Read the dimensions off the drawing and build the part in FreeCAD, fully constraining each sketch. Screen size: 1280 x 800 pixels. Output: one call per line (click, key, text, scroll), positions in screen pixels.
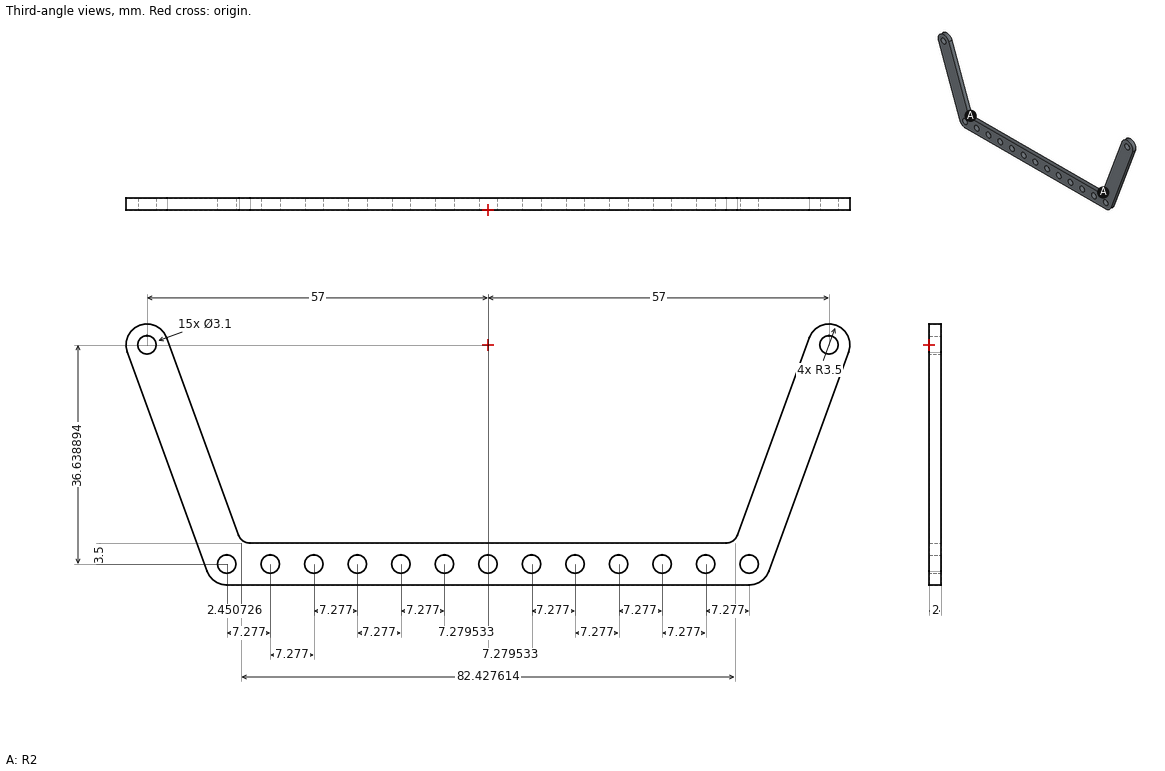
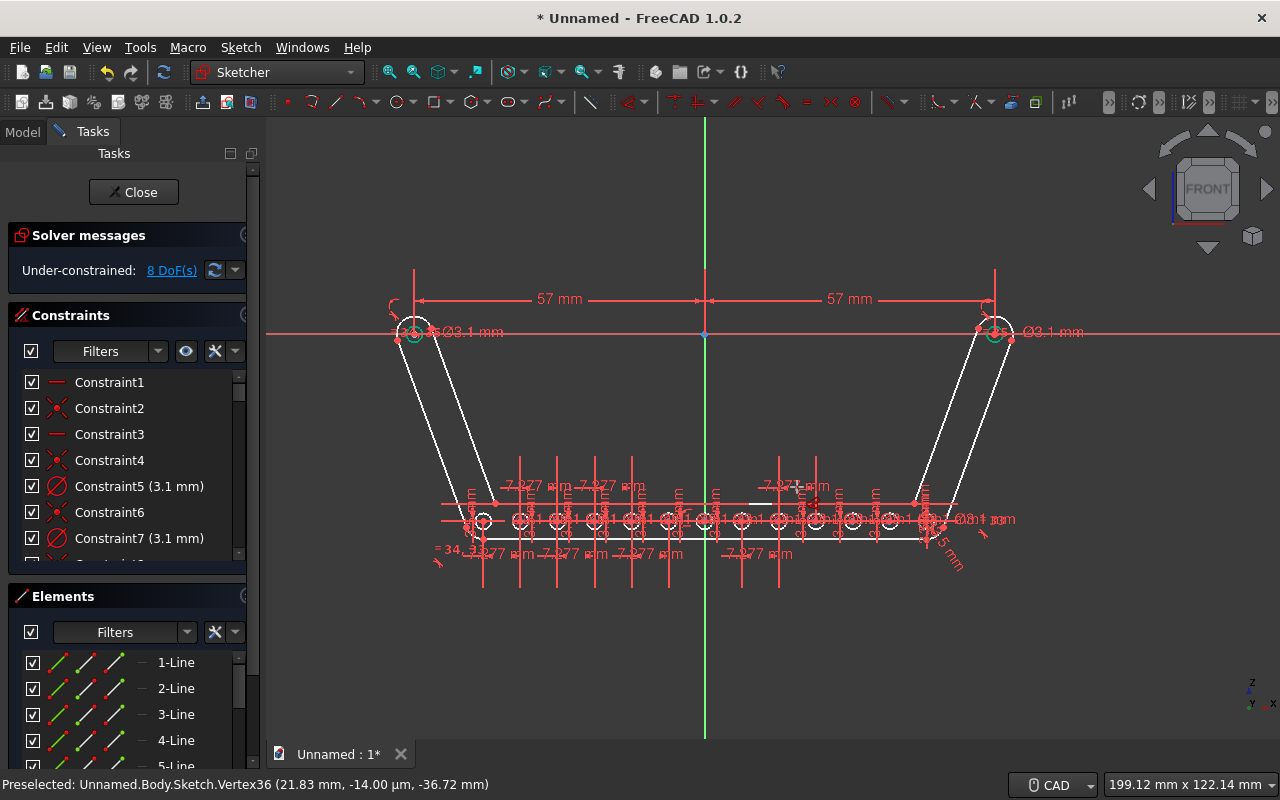
click(816, 521)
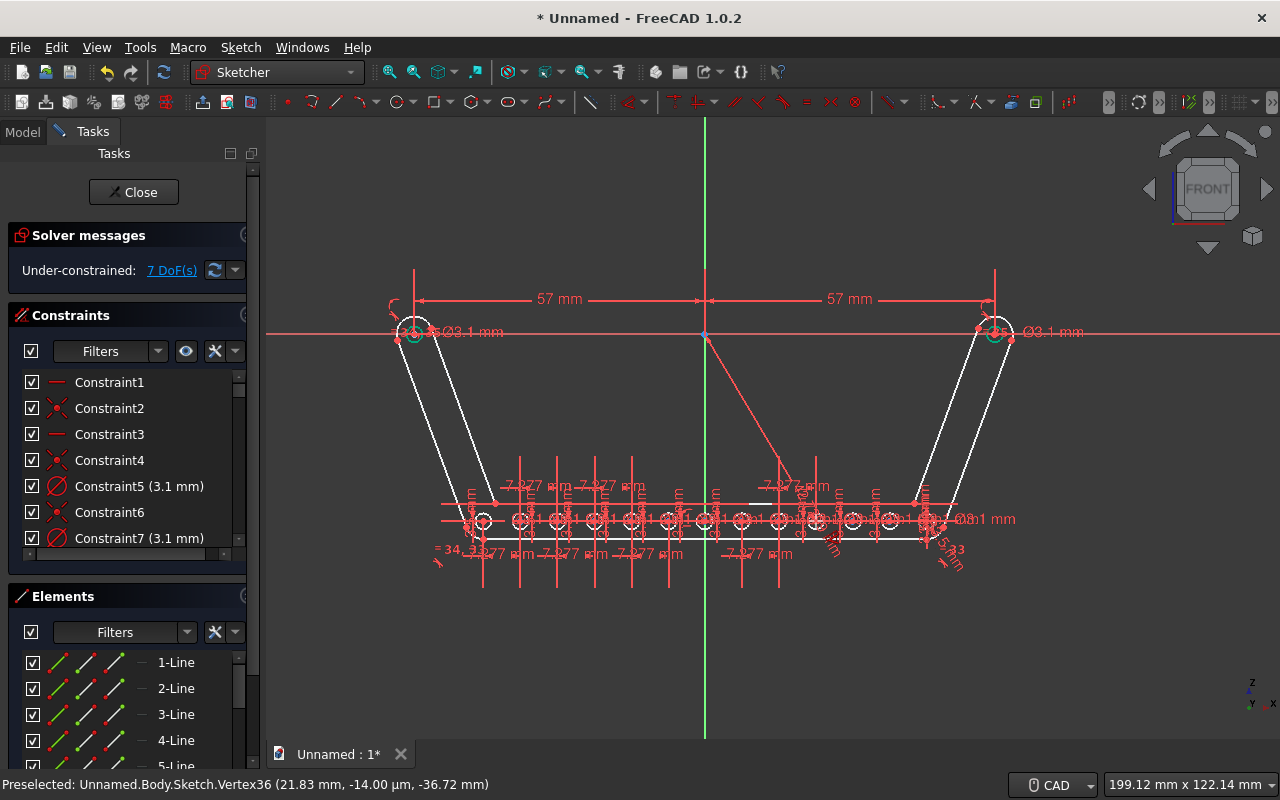
click(853, 521)
click(834, 555)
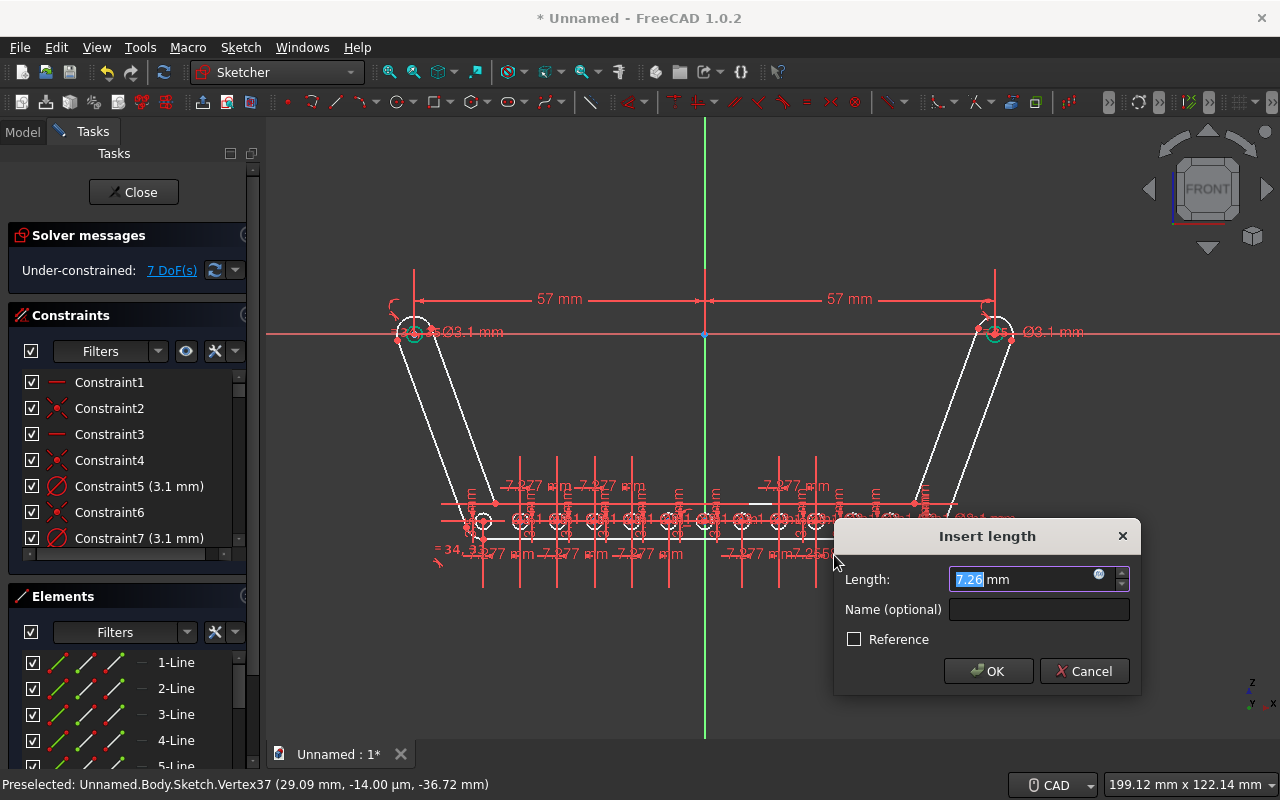
text(7.277)
key(Return)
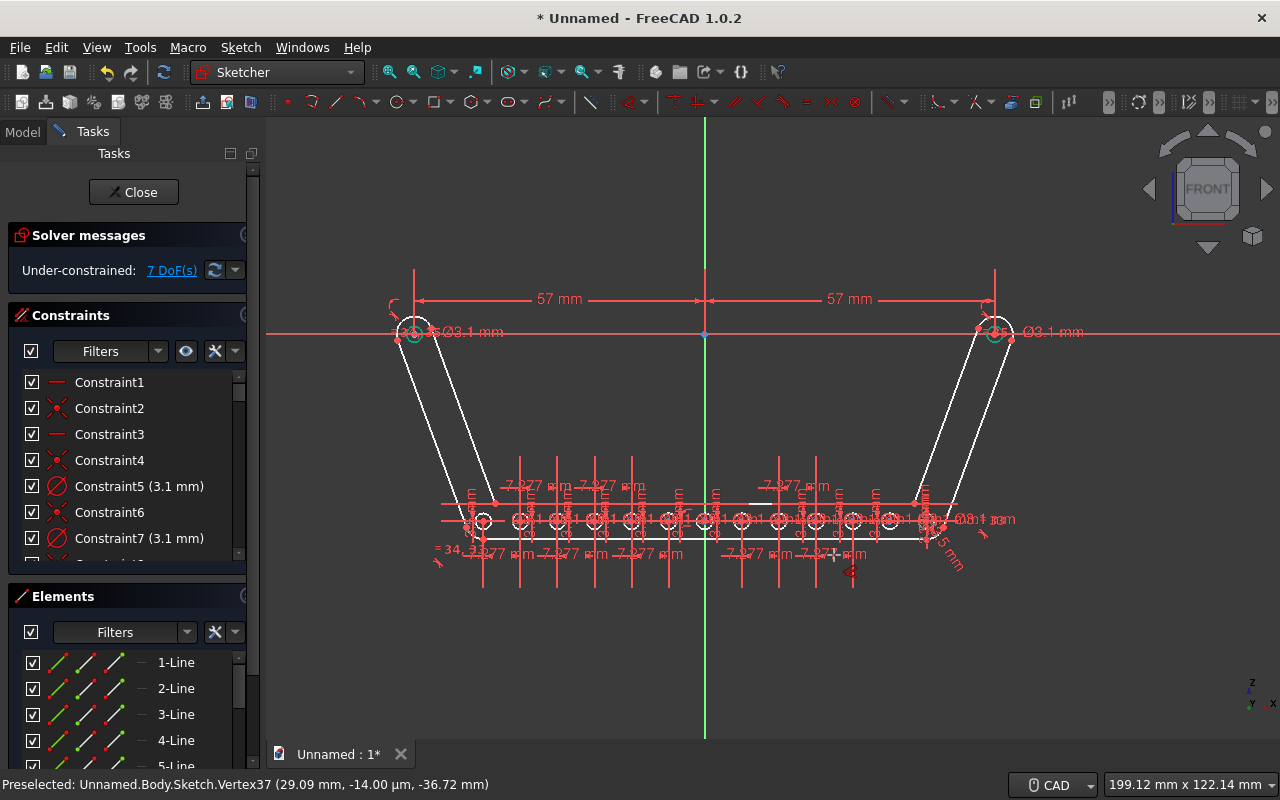
click(853, 521)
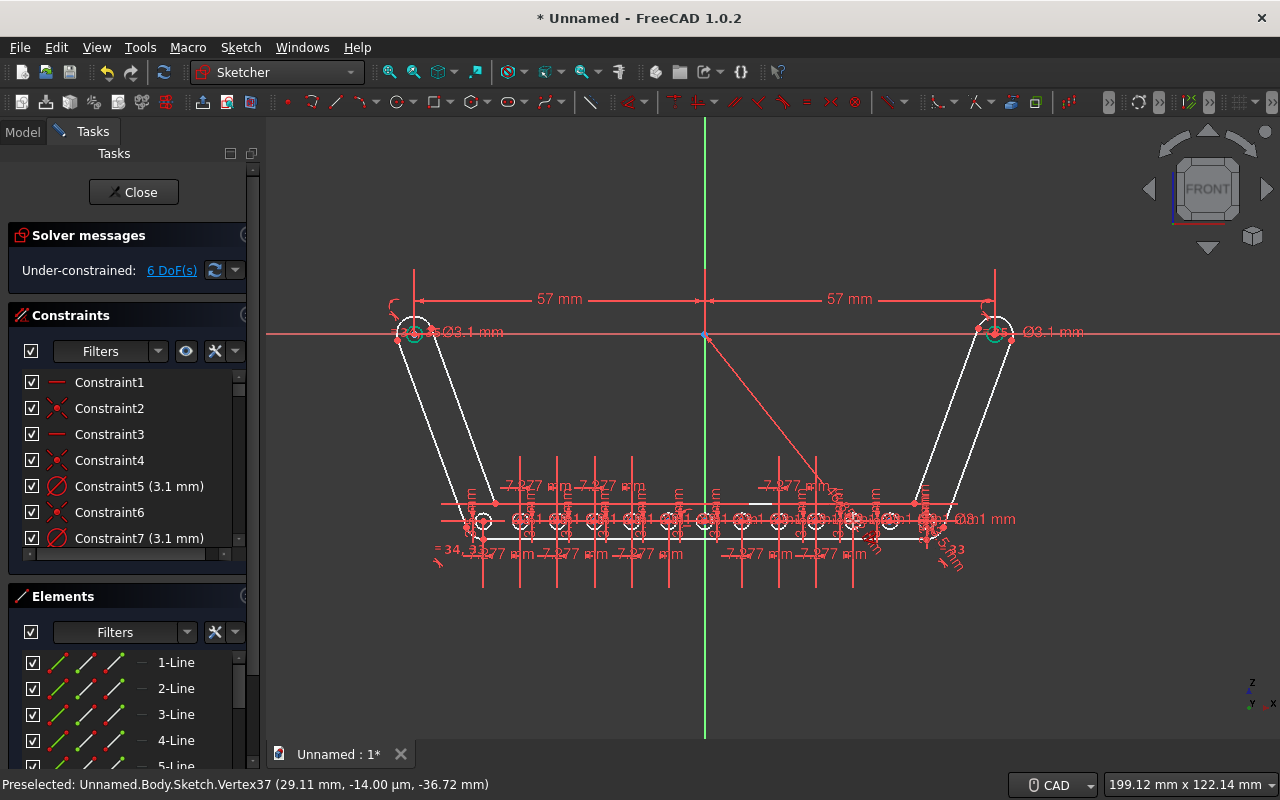
click(890, 521)
click(871, 487)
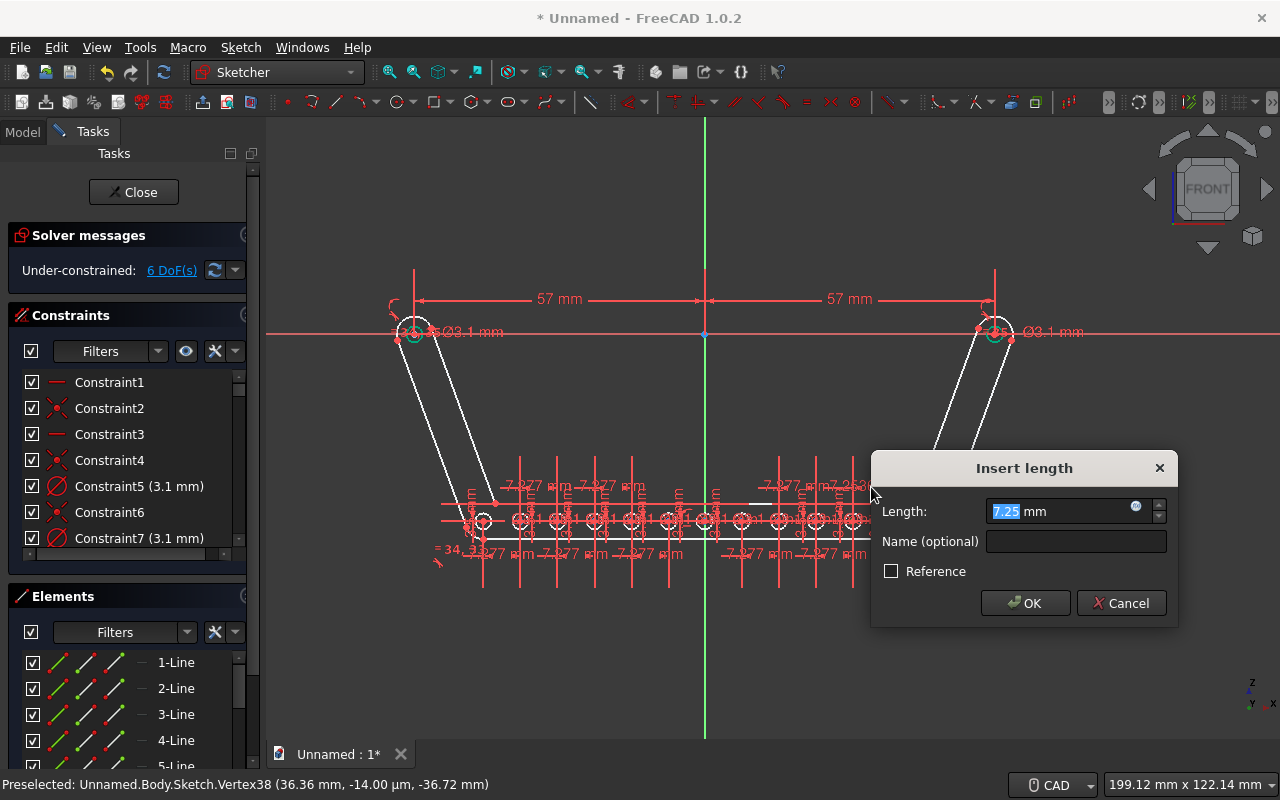
text(7.277)
key(Return)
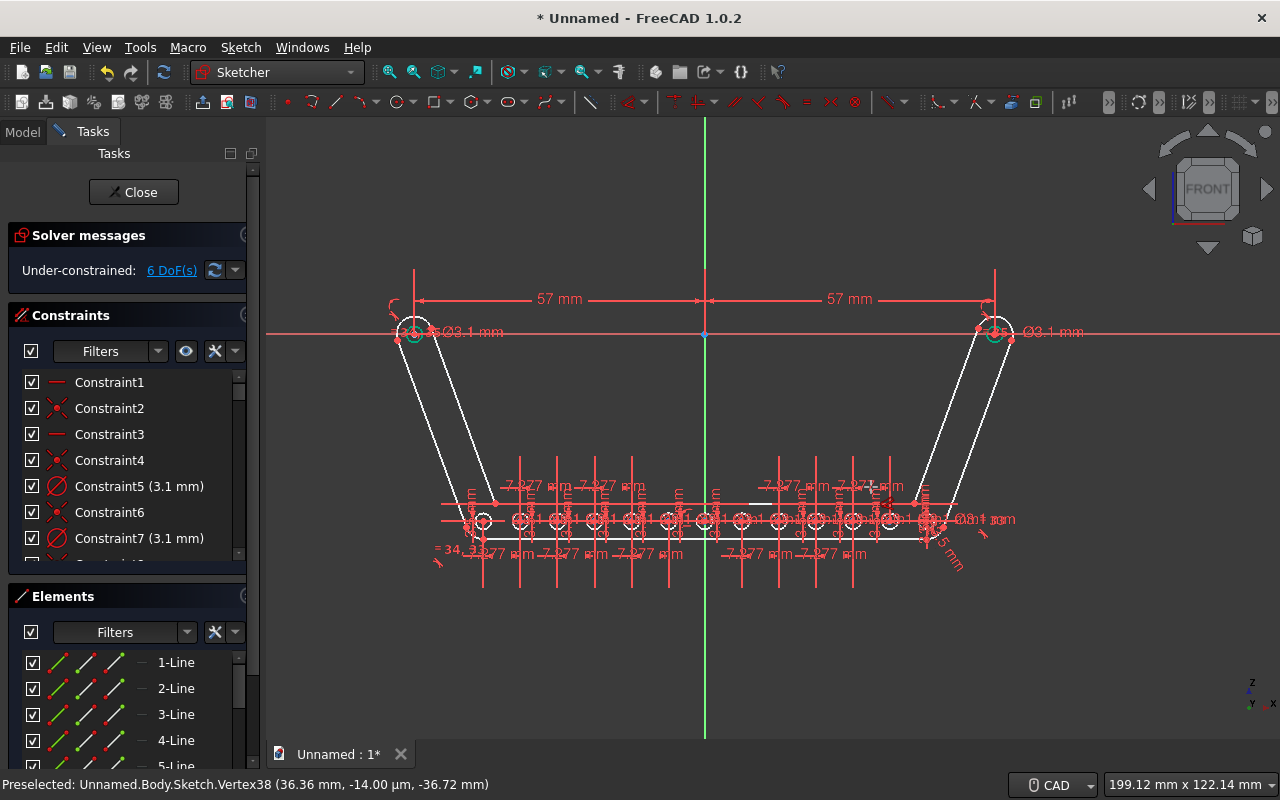
click(927, 539)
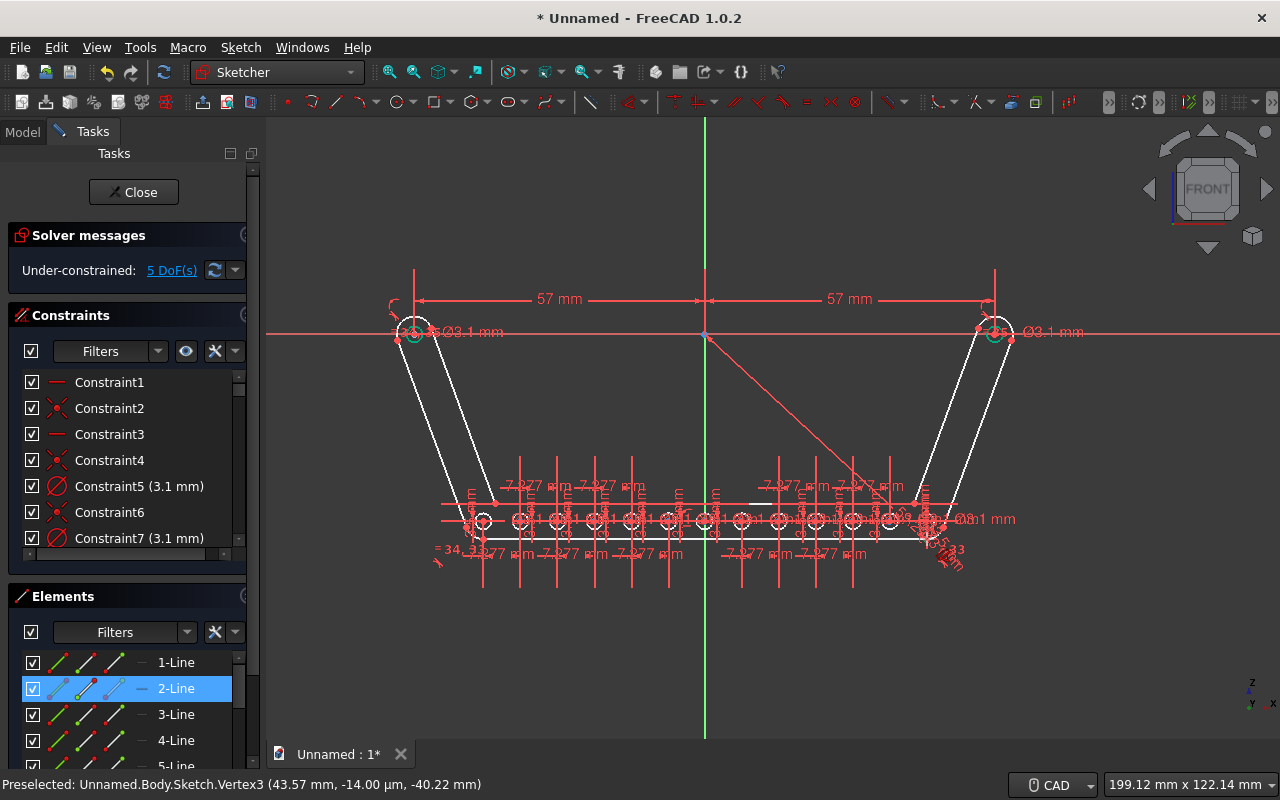
click(890, 521)
click(908, 573)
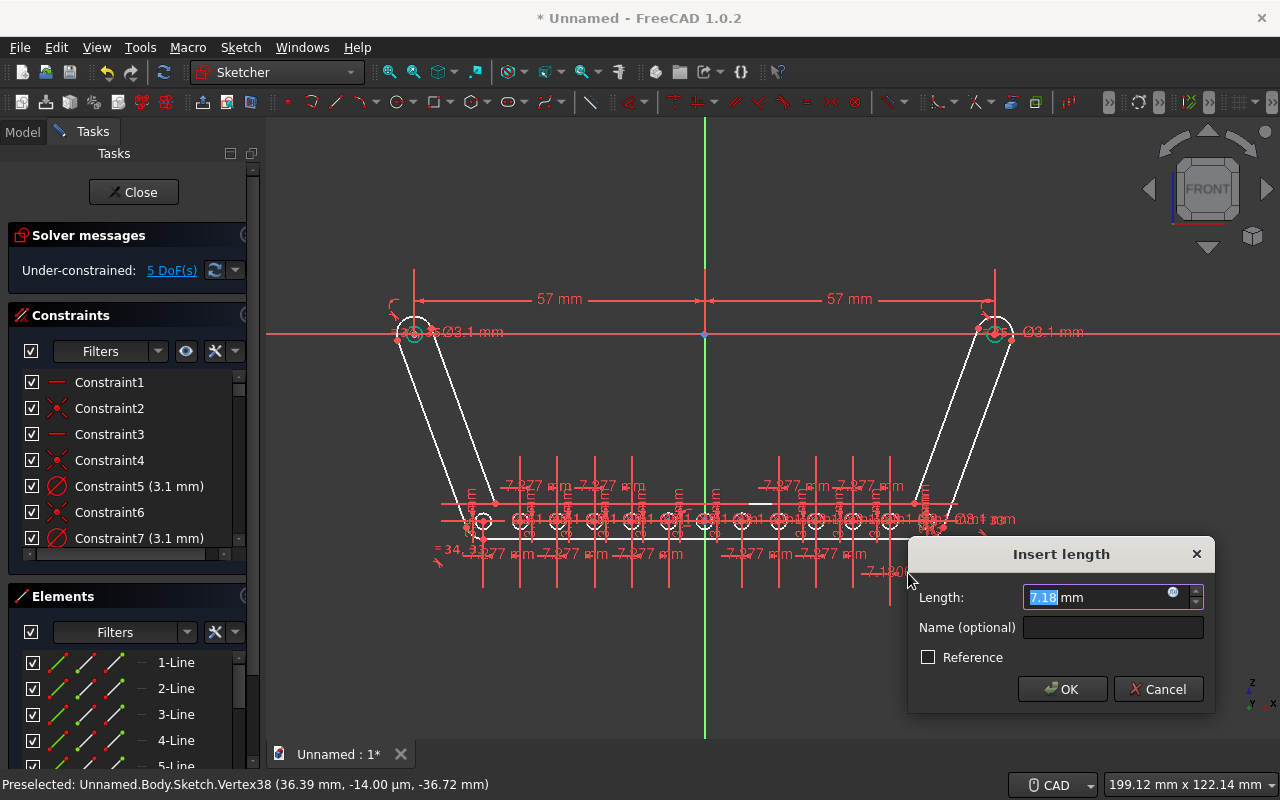
text(7.277)
key(Return)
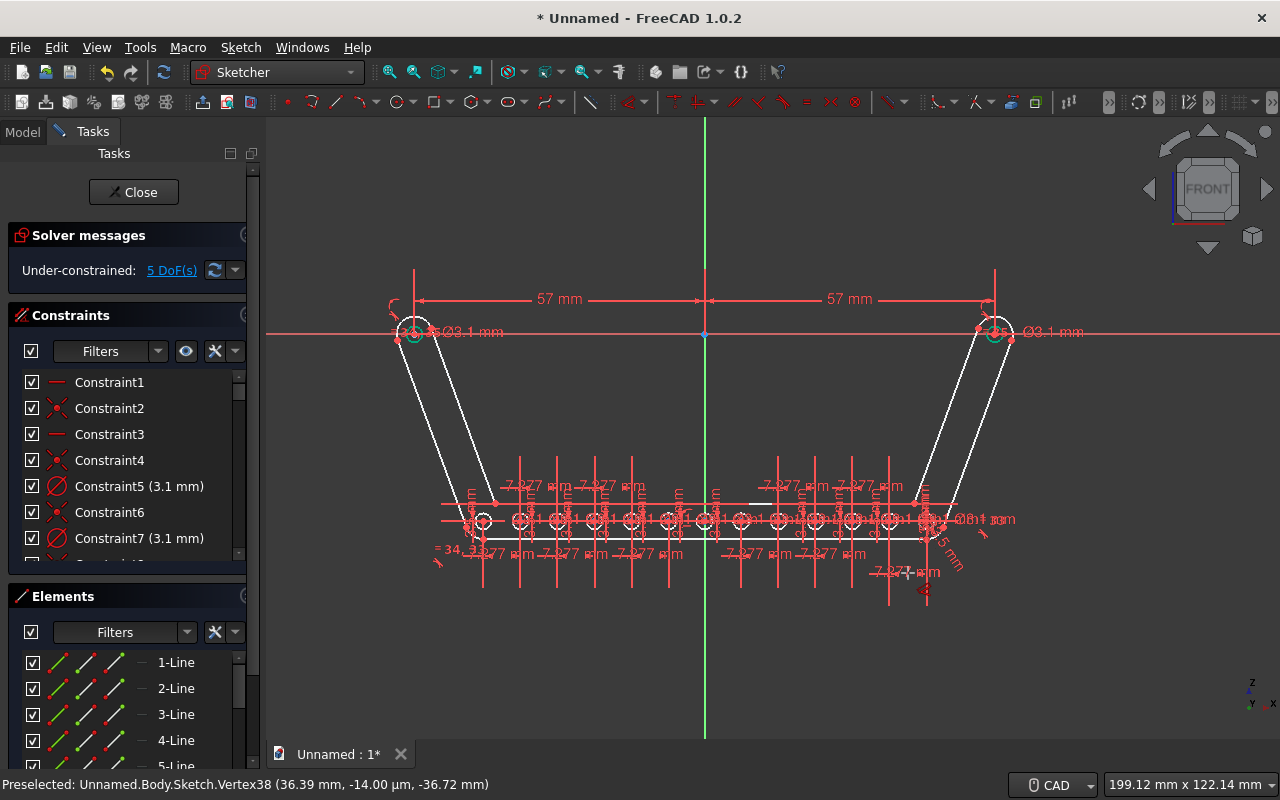
click(669, 521)
click(687, 300)